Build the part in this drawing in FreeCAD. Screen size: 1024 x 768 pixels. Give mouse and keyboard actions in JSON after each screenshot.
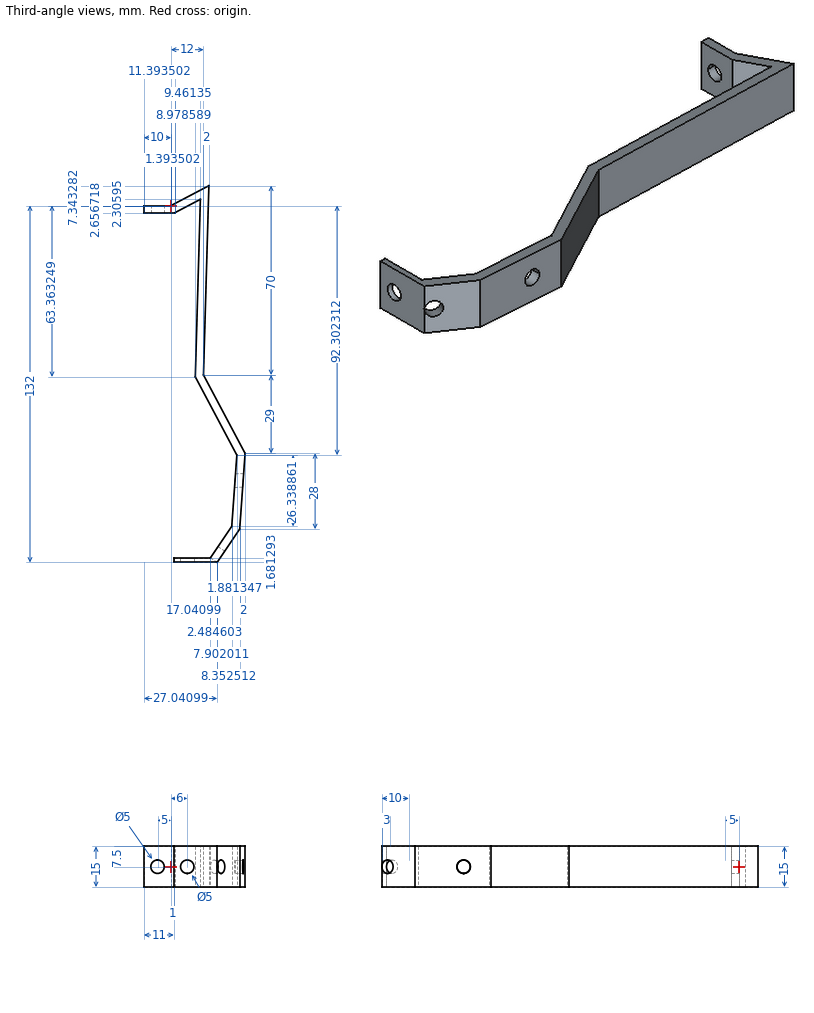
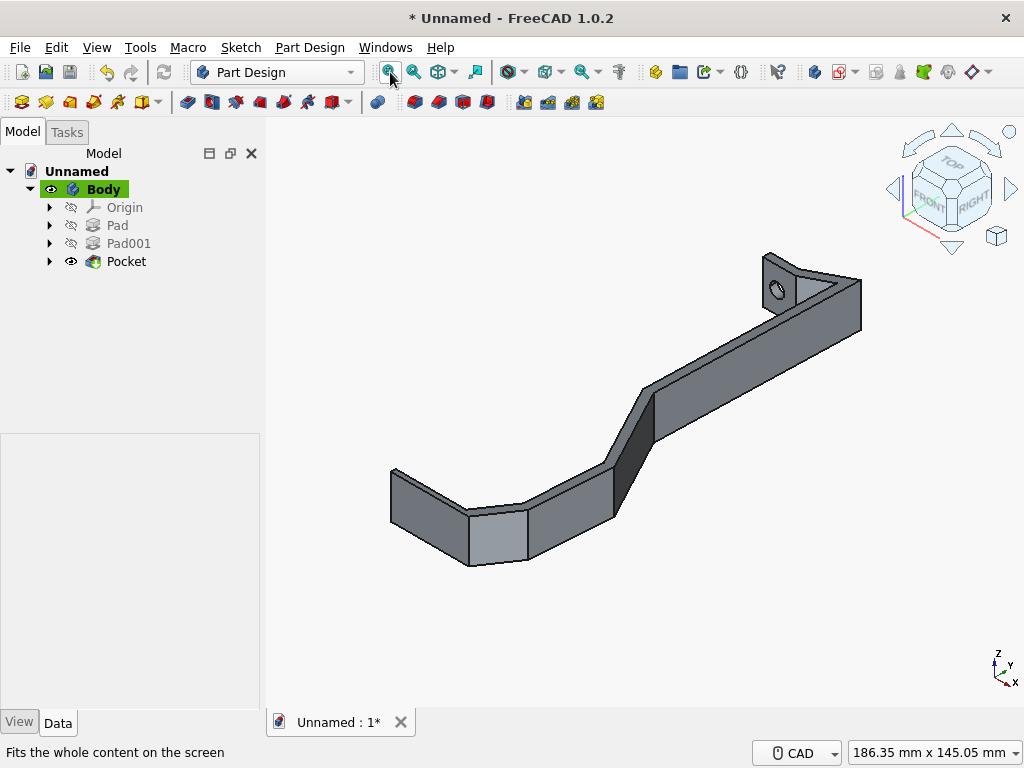
{"action": "left_click", "coordinate": [441, 525]}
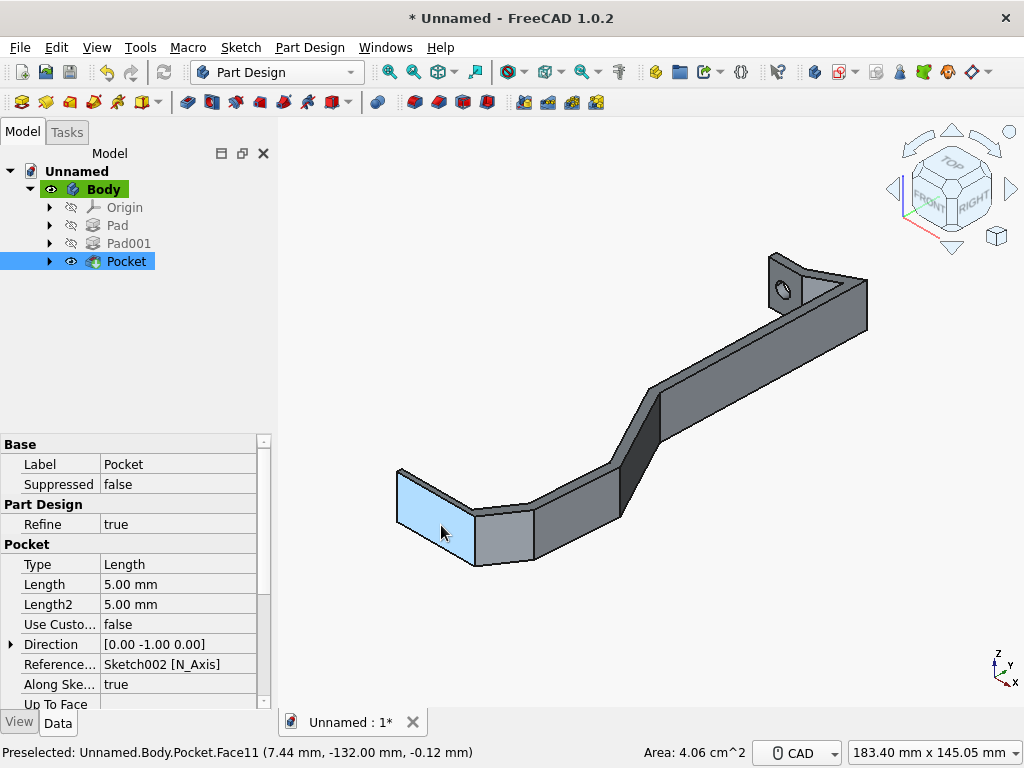
{"action": "left_click", "coordinate": [840, 72]}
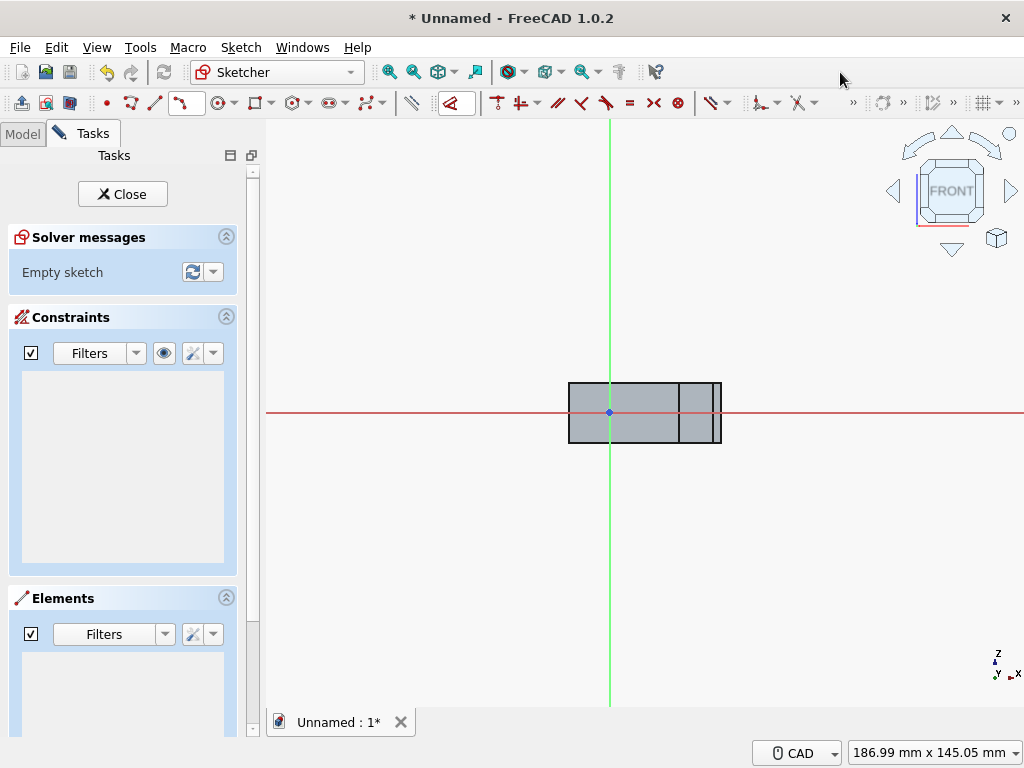
{"action": "scroll", "coordinate": [632, 413], "scroll_direction": "up", "scroll_amount": 12}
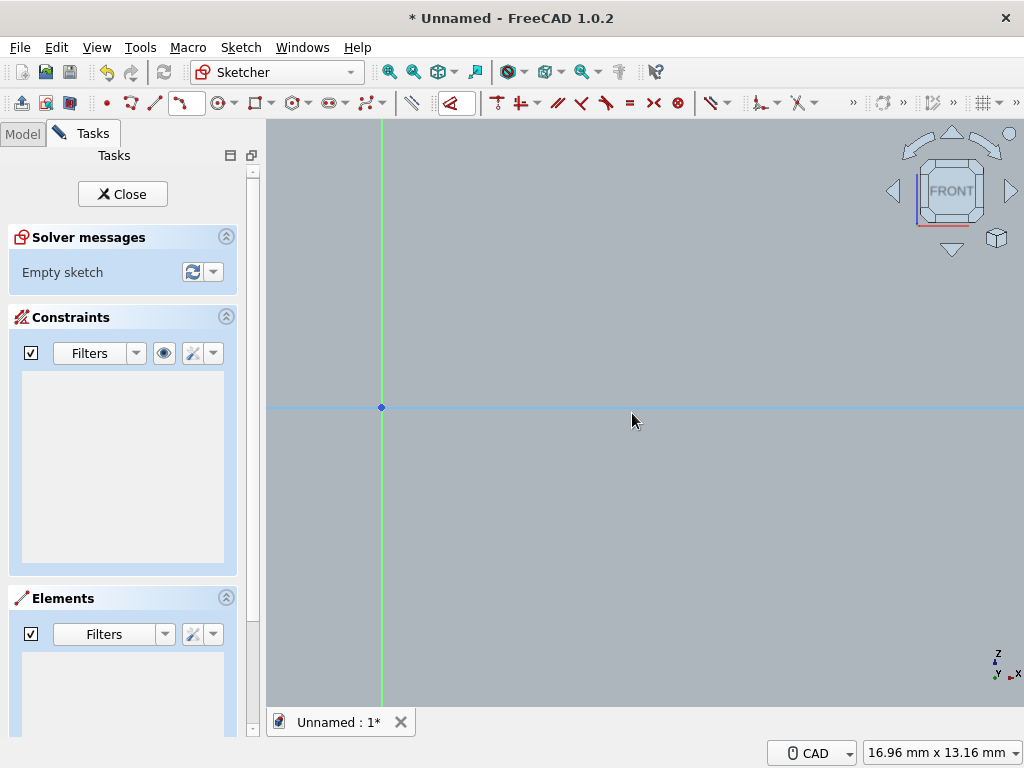
{"action": "left_click", "coordinate": [218, 104]}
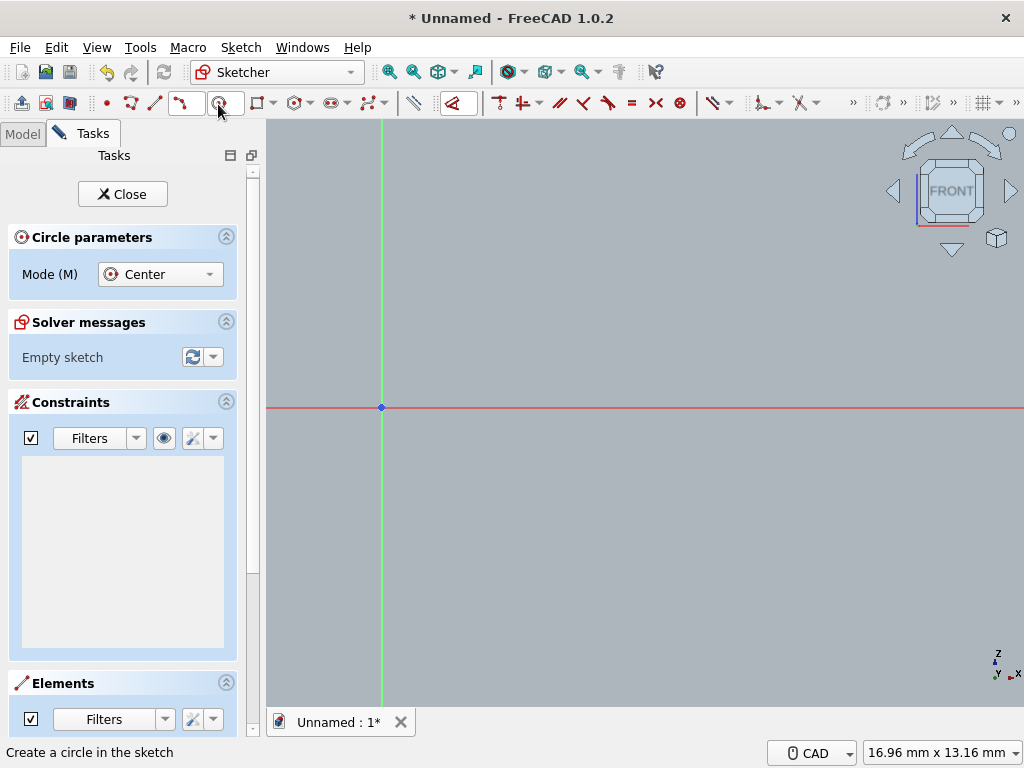
{"action": "left_click", "coordinate": [650, 408]}
{"action": "mouse_move", "coordinate": [729, 329]}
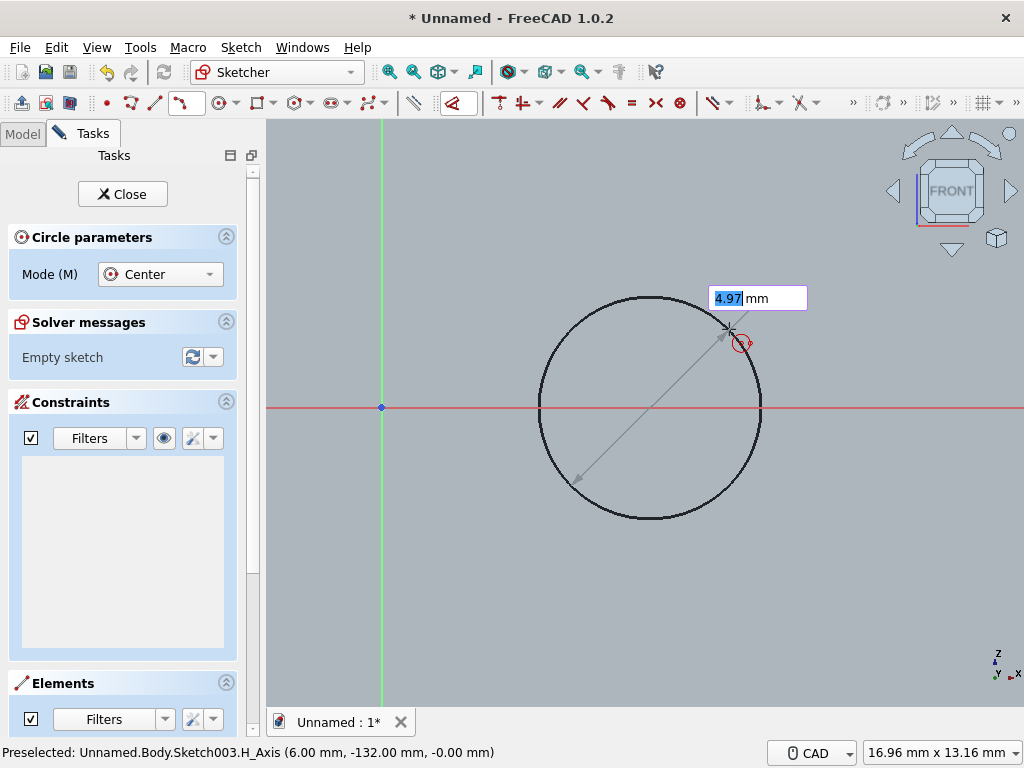
{"action": "type", "text": "5"}
{"action": "key", "text": "Return"}
{"action": "key", "text": "Escape"}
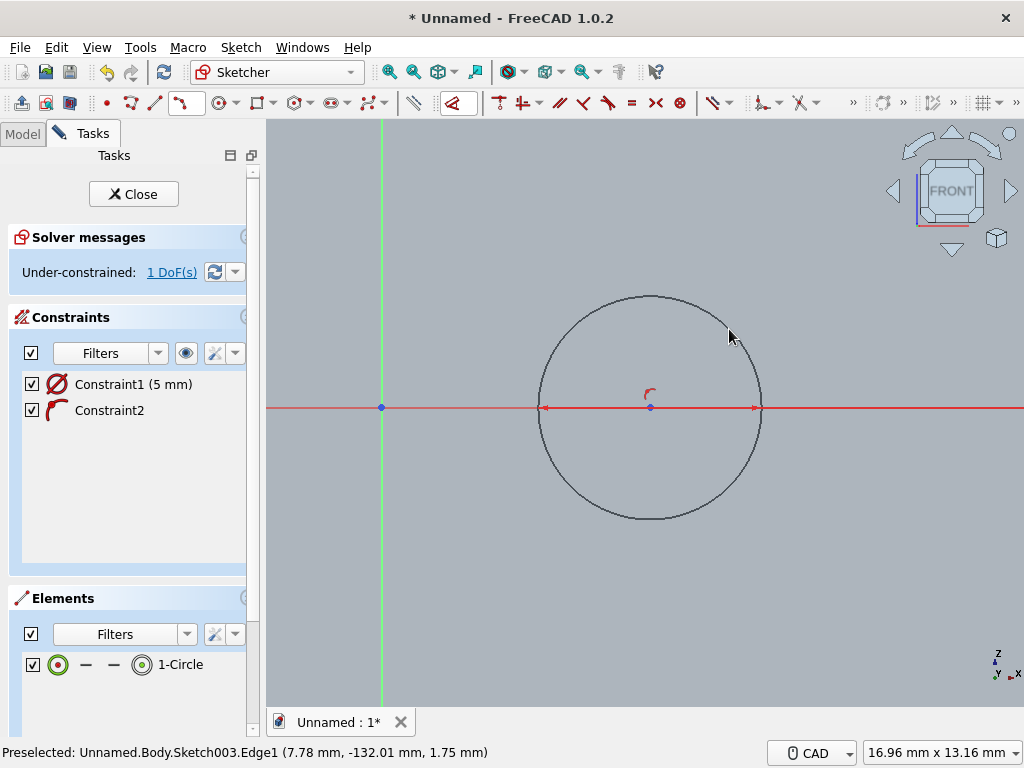
{"action": "left_click", "coordinate": [650, 408]}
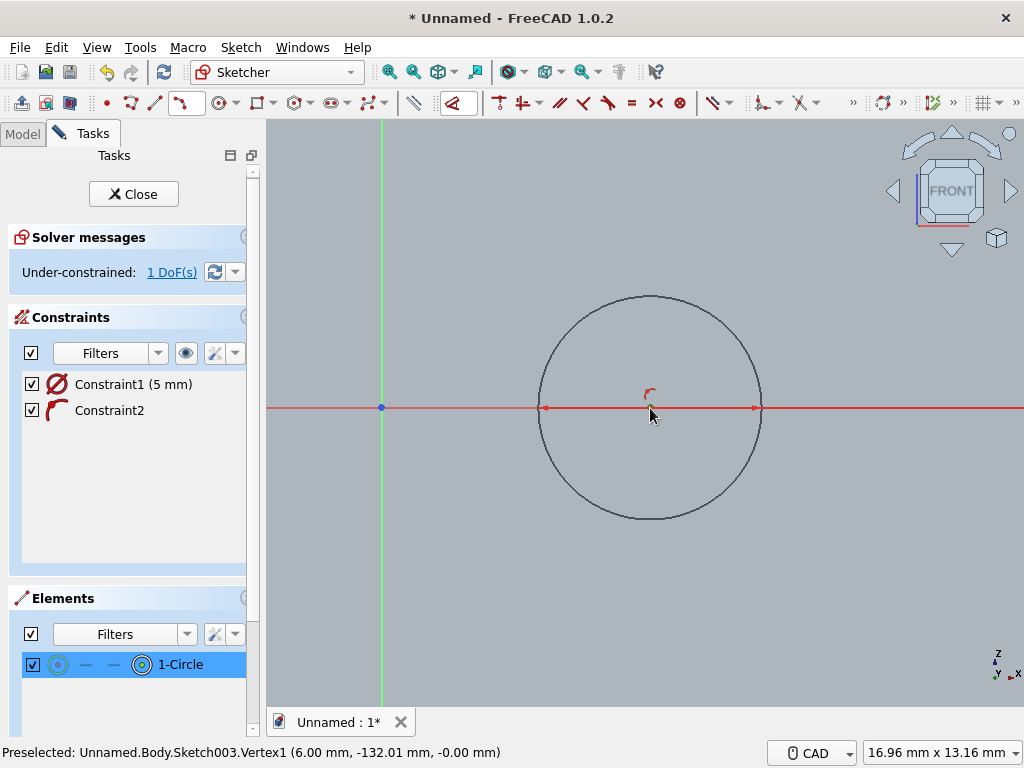
{"action": "key", "text": "l"}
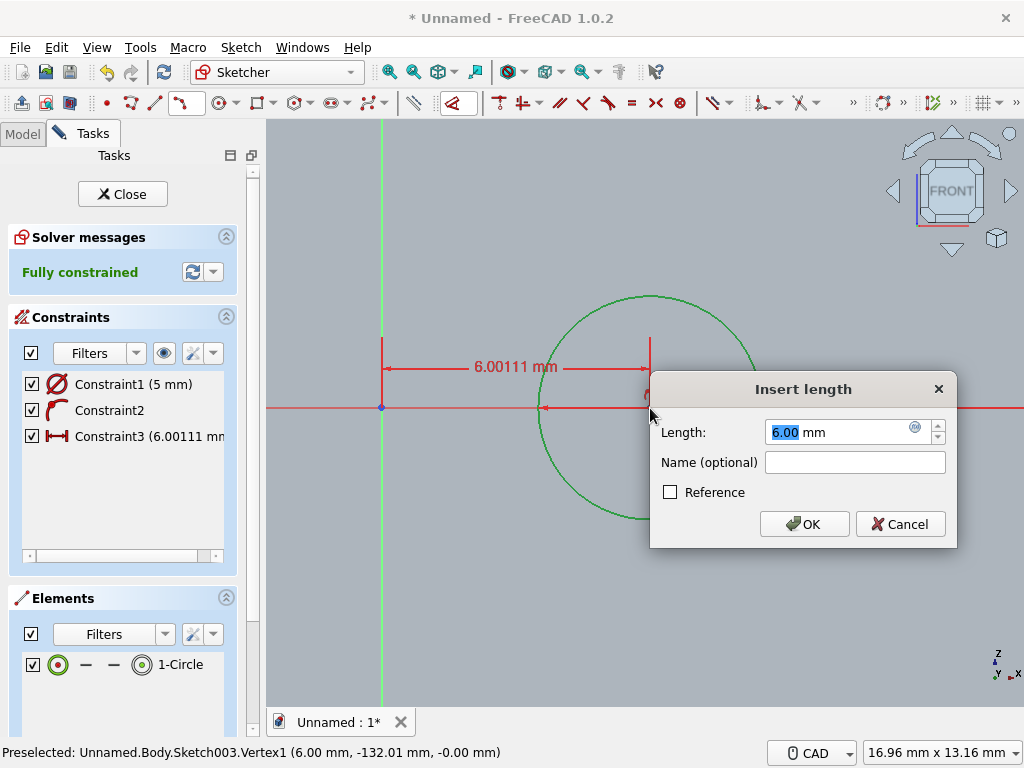
{"action": "type", "text": "6"}
{"action": "key", "text": "Return"}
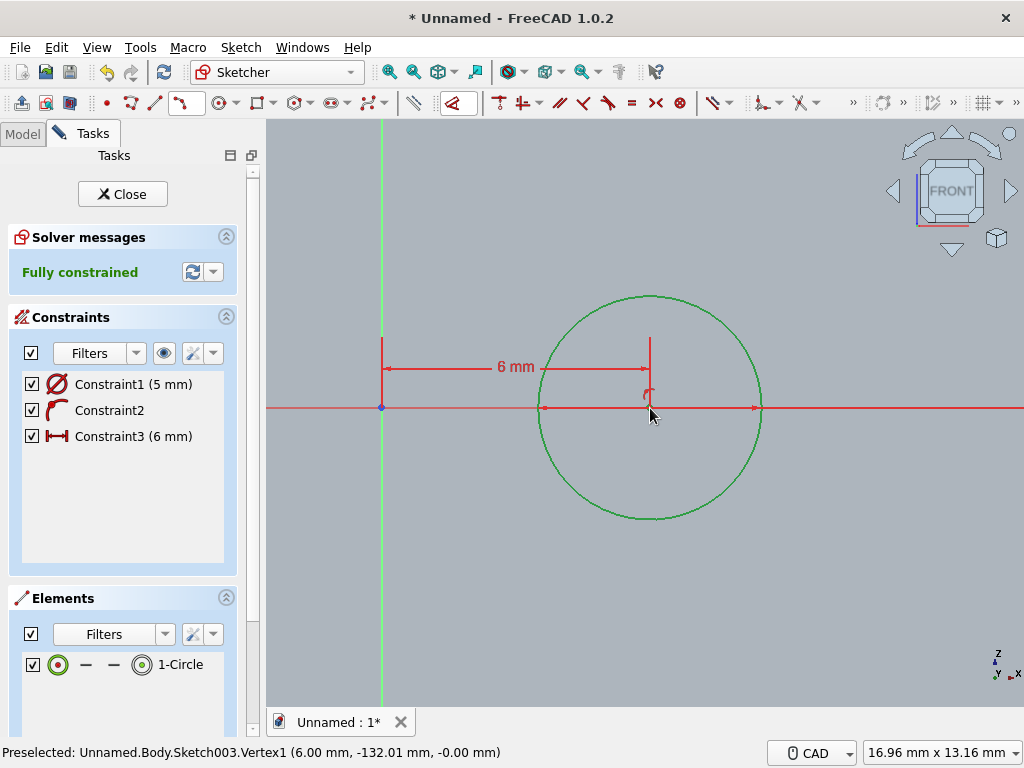
{"action": "left_click", "coordinate": [123, 194]}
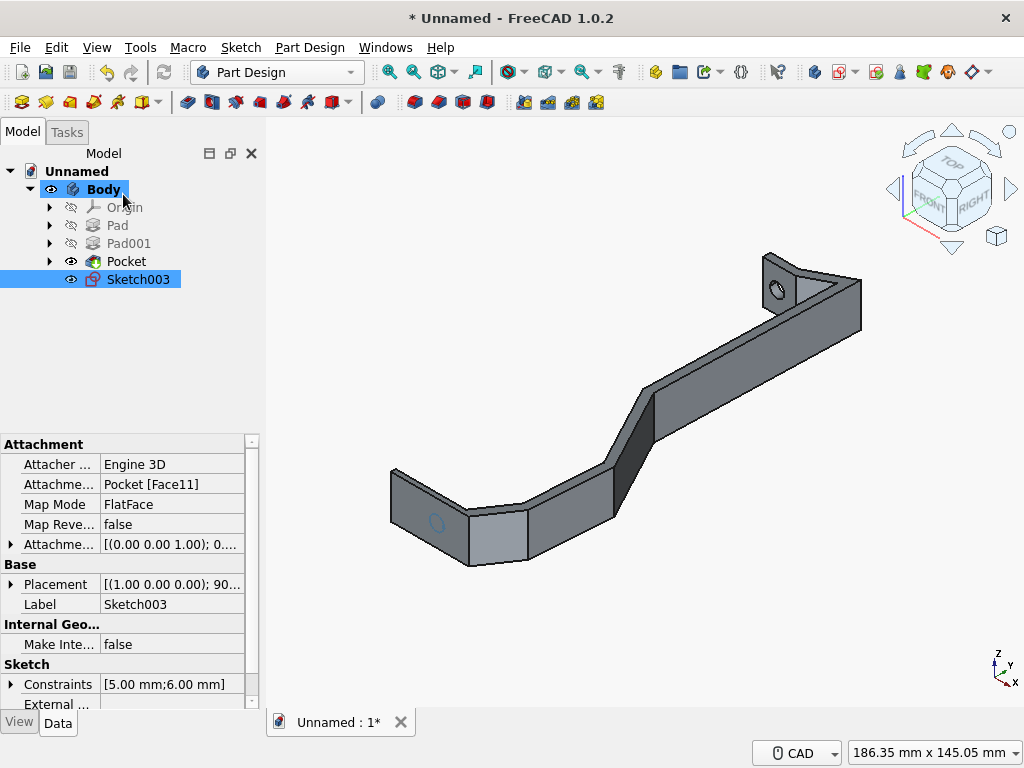
{"action": "left_click", "coordinate": [188, 102]}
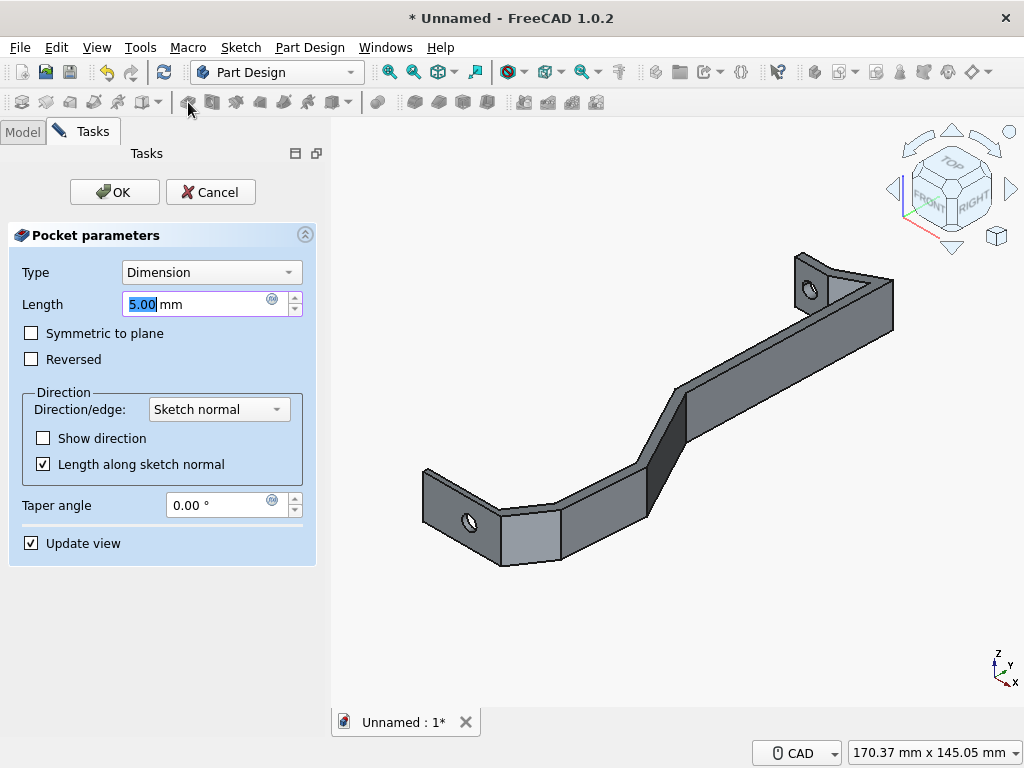
{"action": "type", "text": "10"}
{"action": "key", "text": "Tab"}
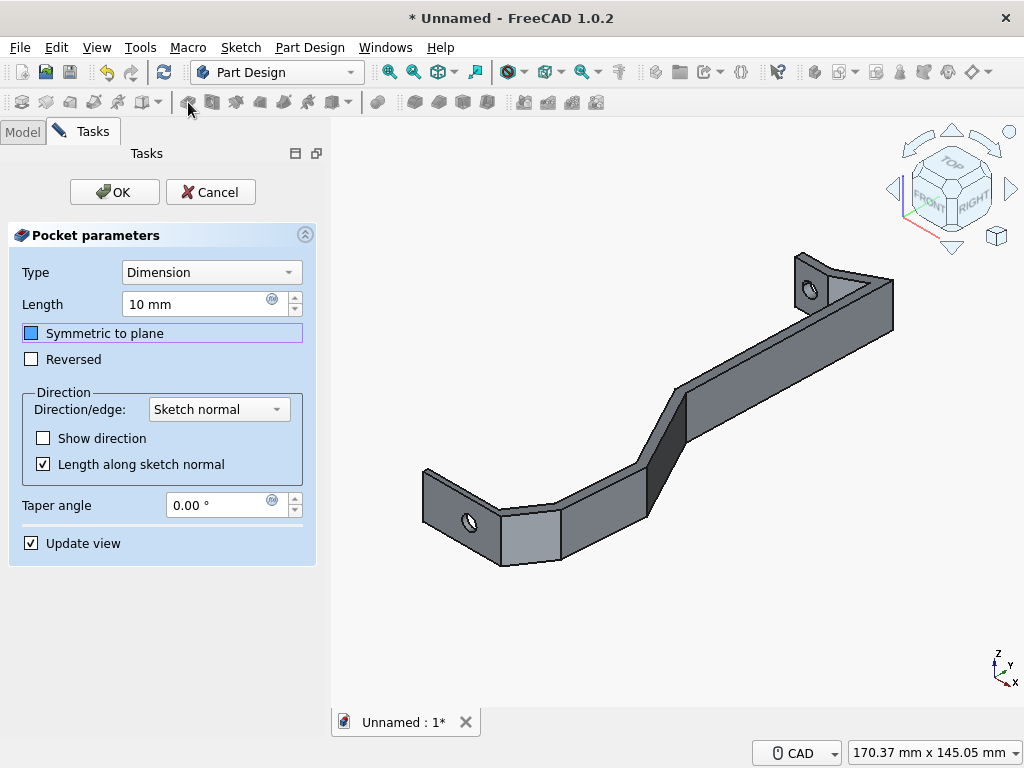
{"action": "left_click", "coordinate": [115, 192]}